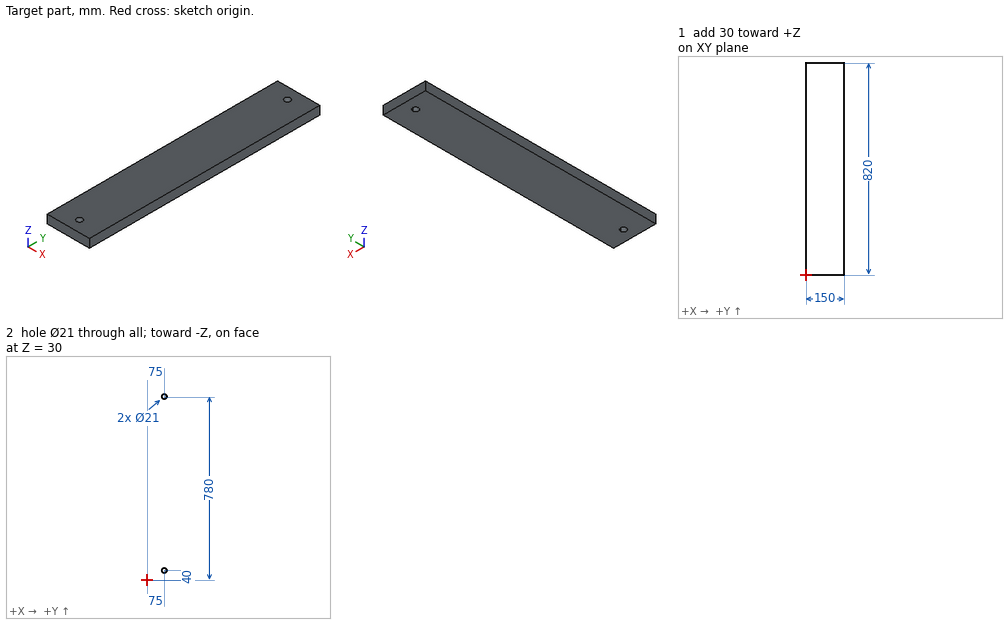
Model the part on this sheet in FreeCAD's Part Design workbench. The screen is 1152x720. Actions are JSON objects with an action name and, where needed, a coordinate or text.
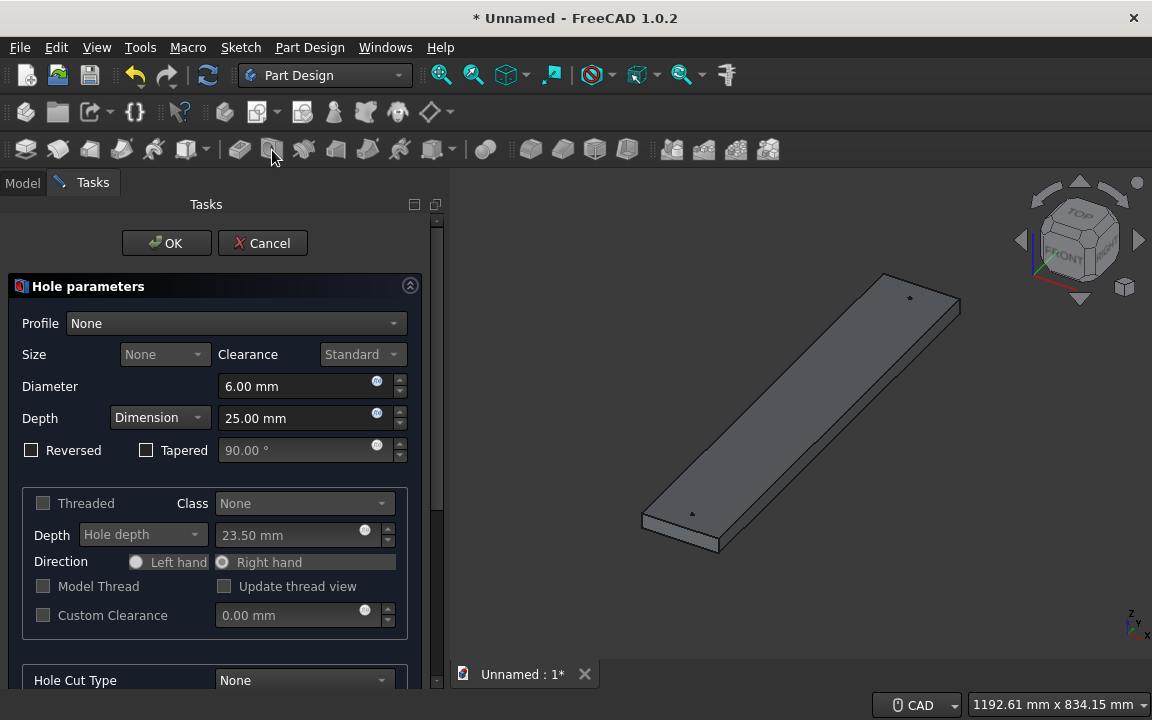
{"action": "triple_click", "coordinate": [305, 386]}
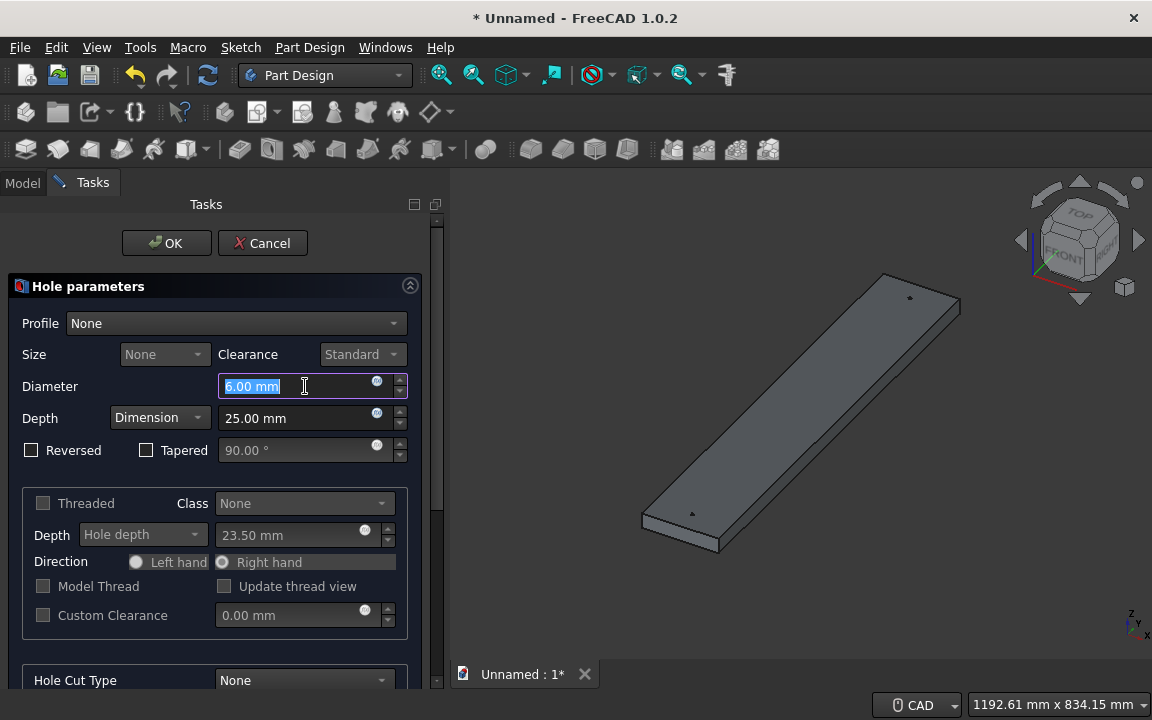
{"action": "type", "text": "21"}
{"action": "key", "text": "Tab"}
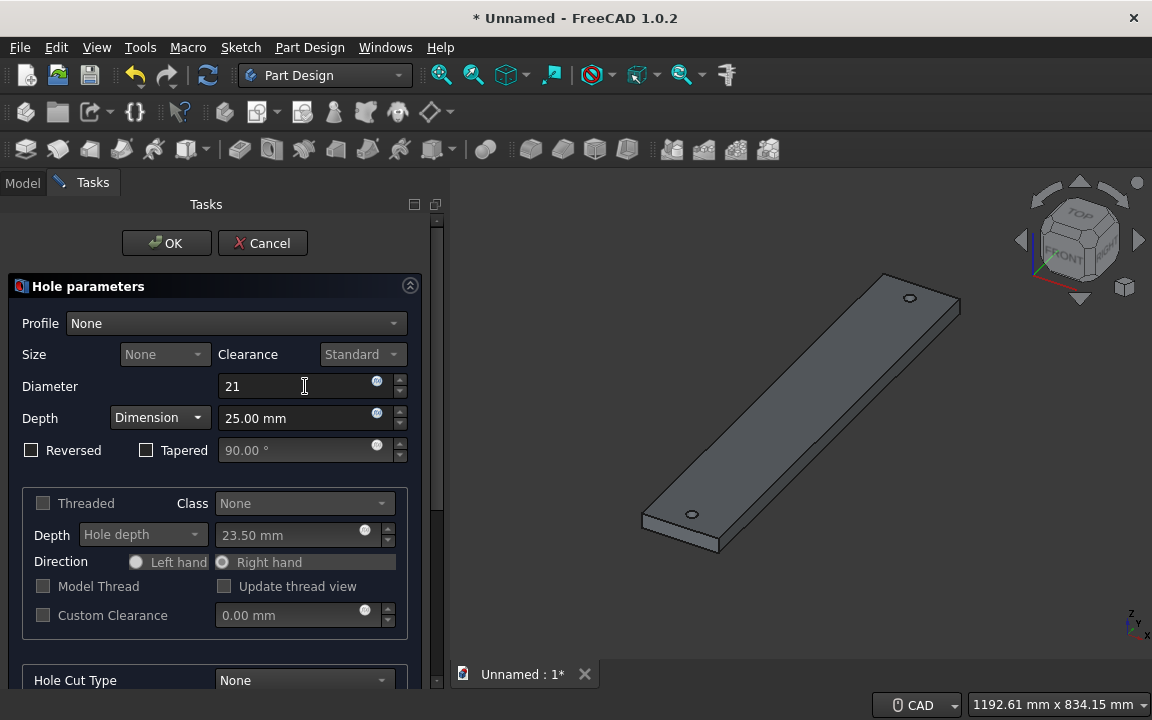
{"action": "left_click", "coordinate": [161, 418]}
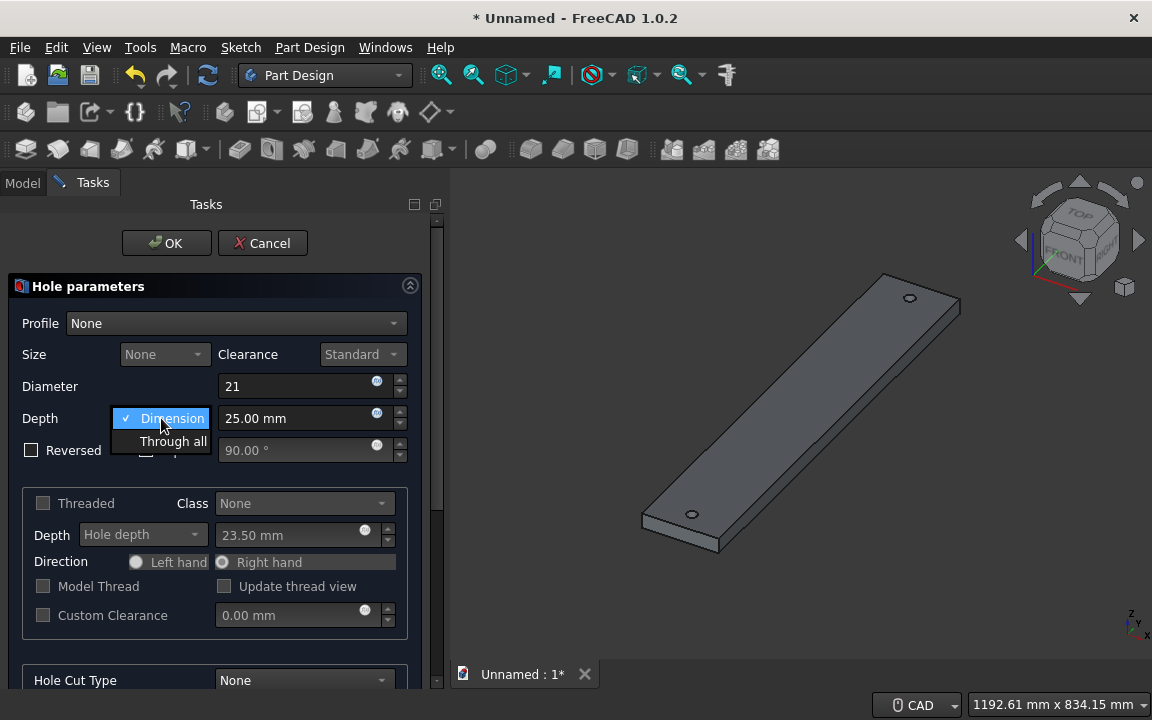
{"action": "left_click", "coordinate": [160, 442]}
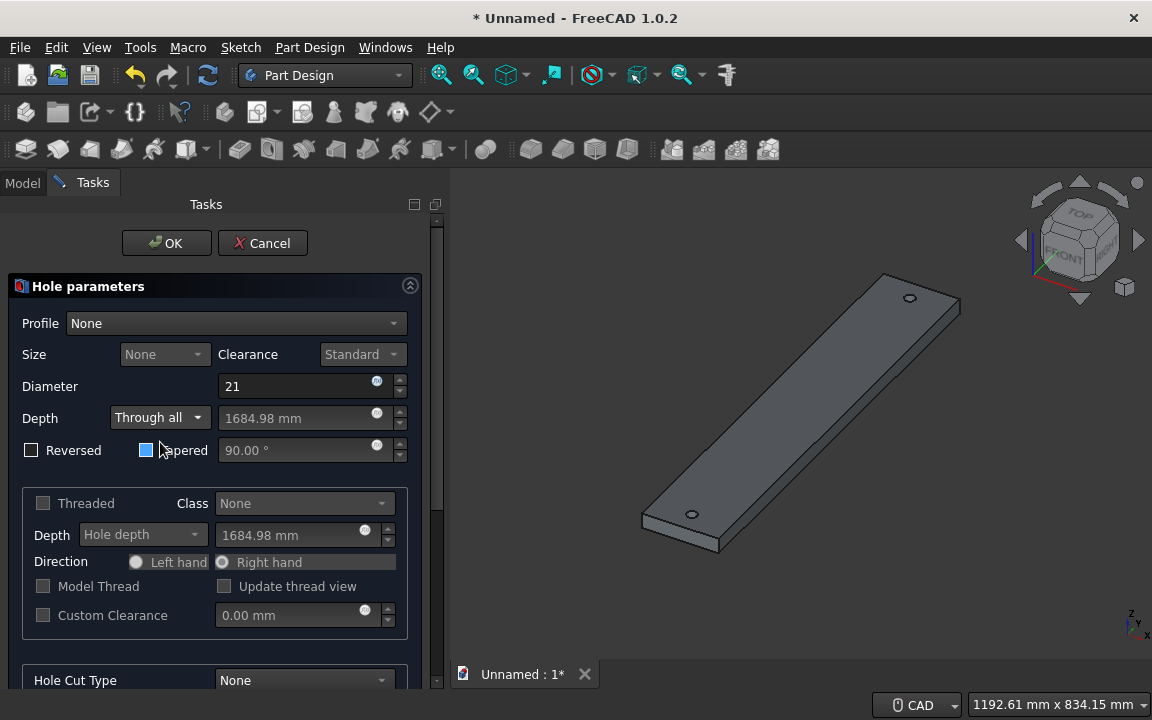
{"action": "left_click", "coordinate": [167, 243]}